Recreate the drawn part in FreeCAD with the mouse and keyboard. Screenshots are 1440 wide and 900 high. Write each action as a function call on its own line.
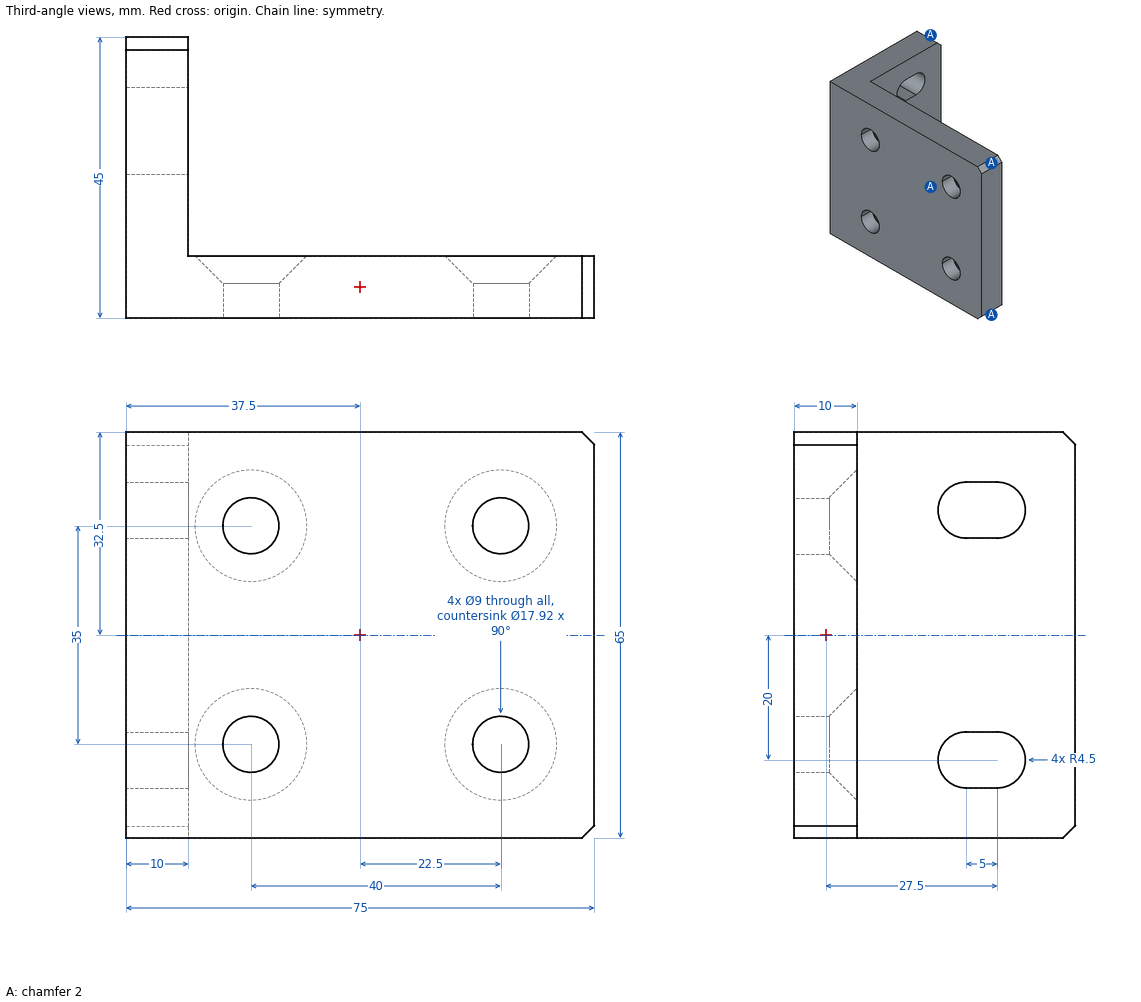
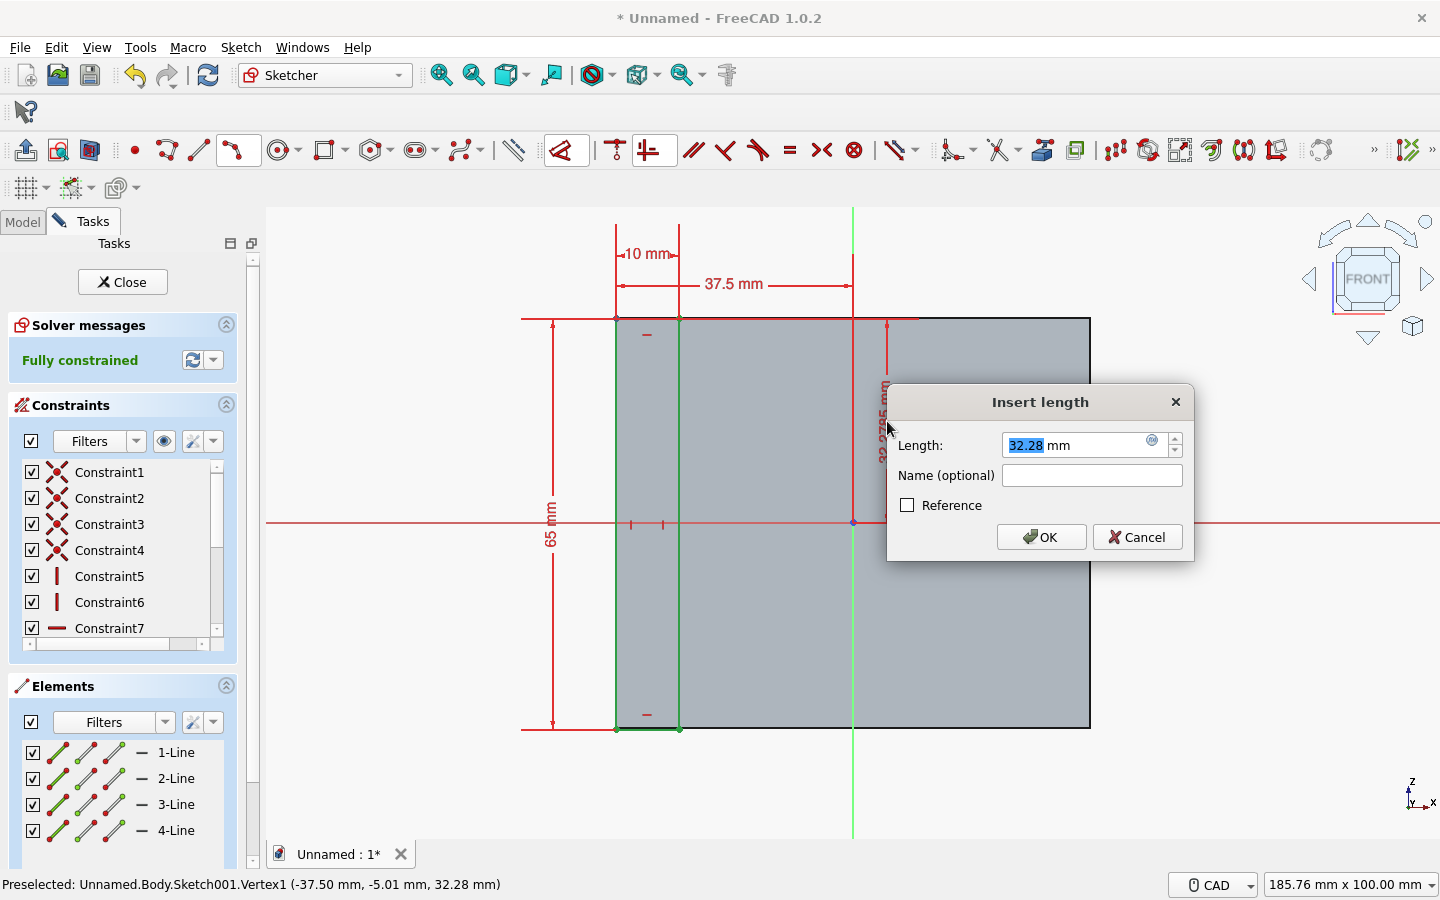
text(32.5)
key(Return)
key(Escape)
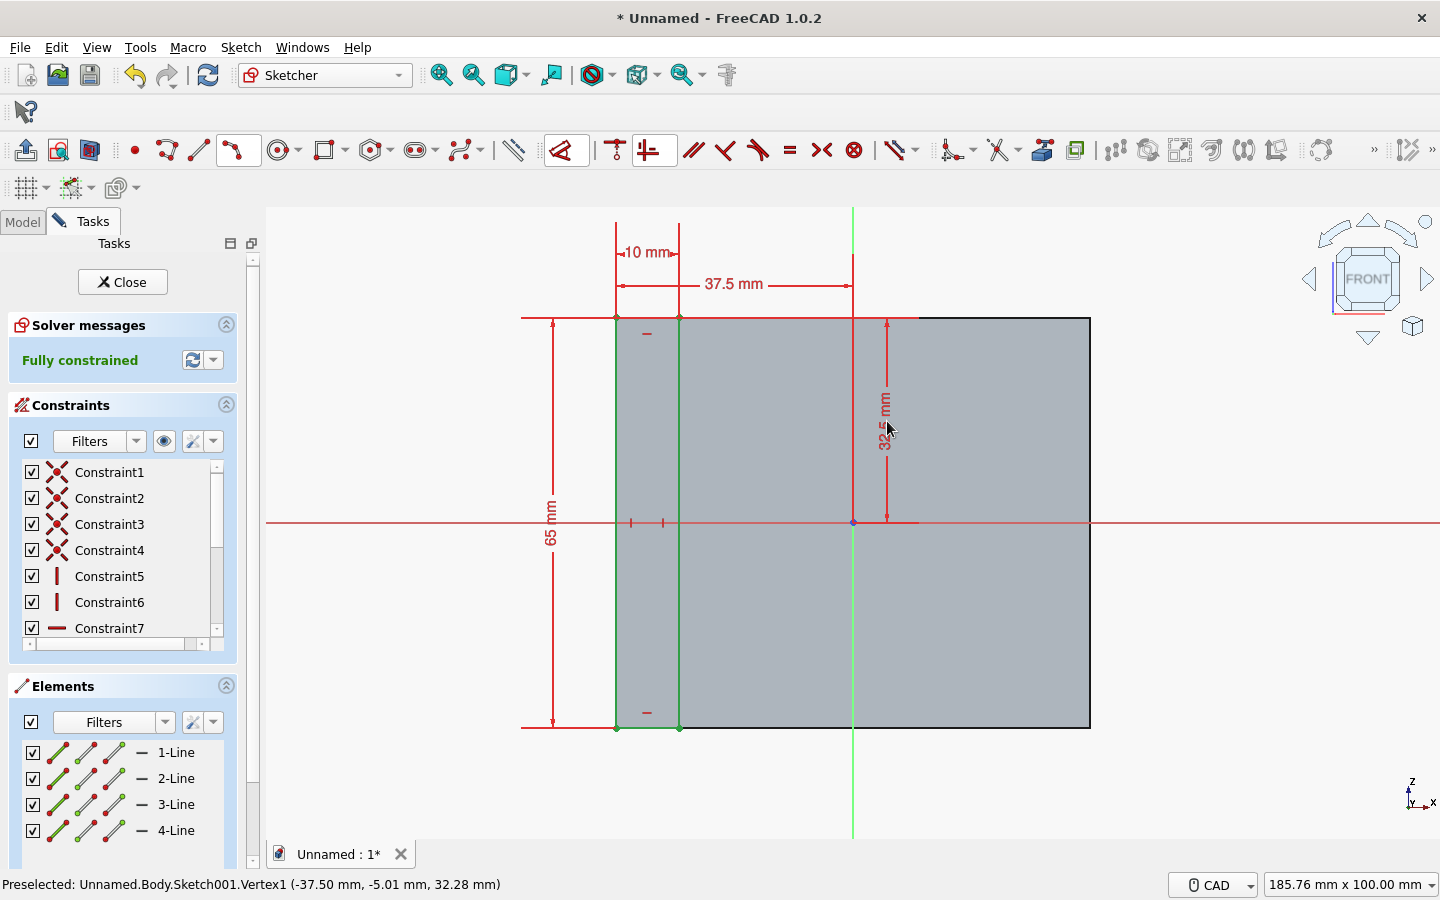
click(123, 282)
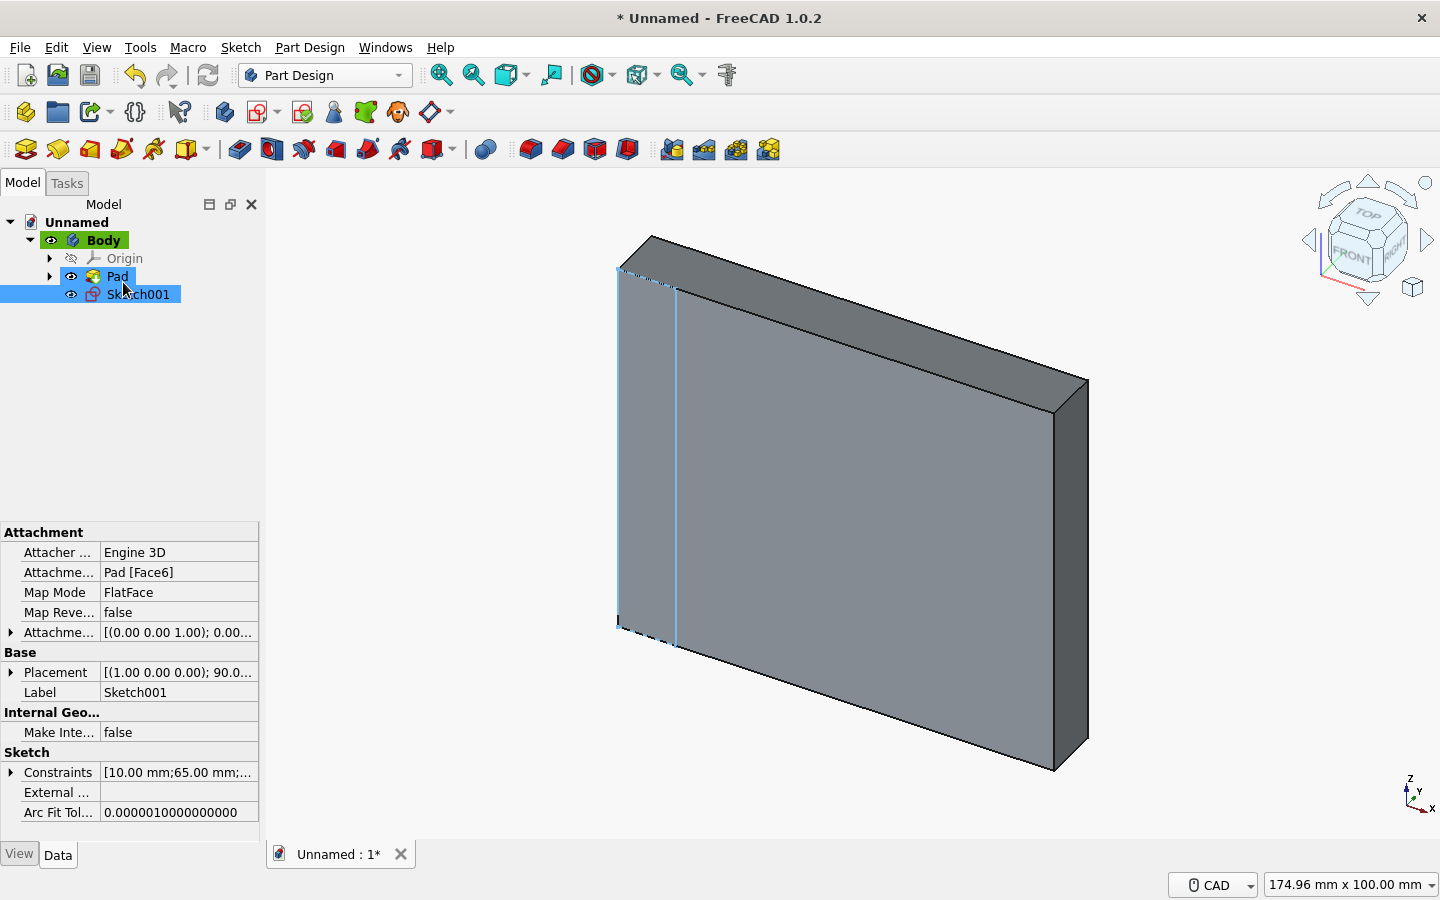
click(26, 150)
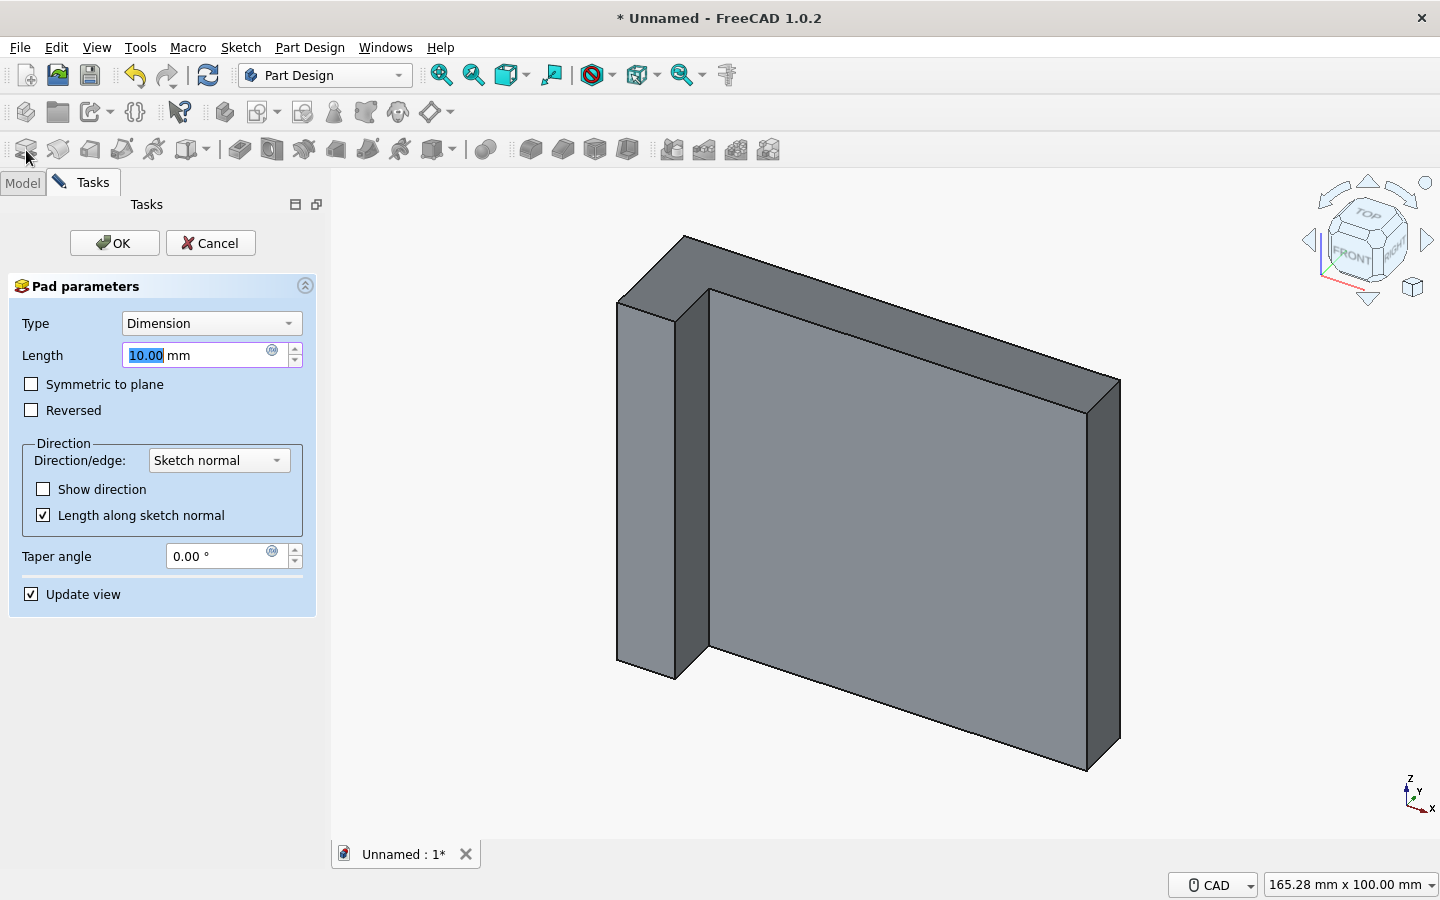
text(45)
key(Tab)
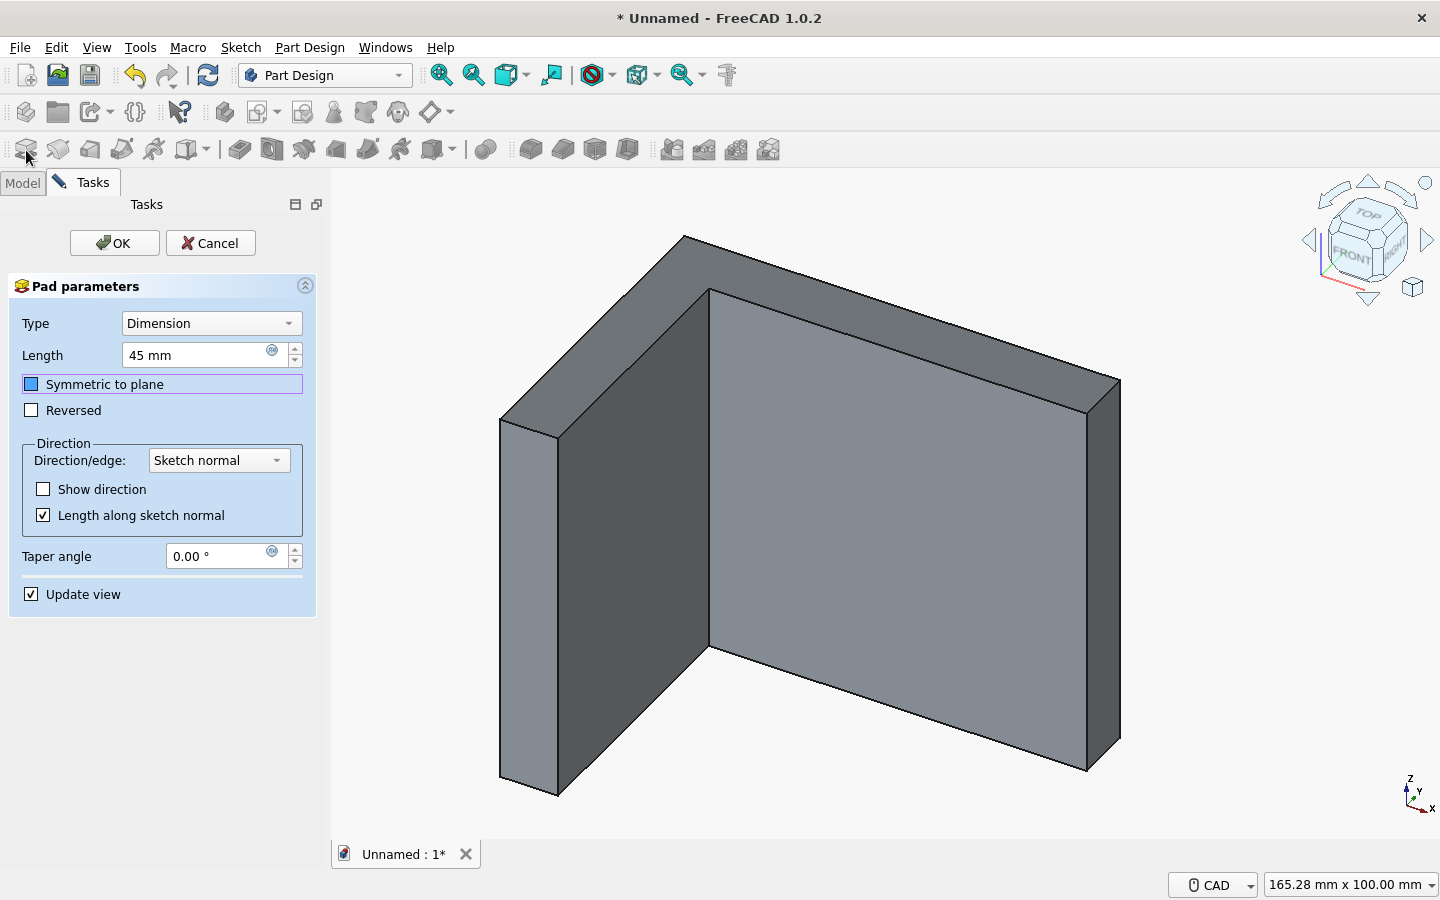
click(30, 410)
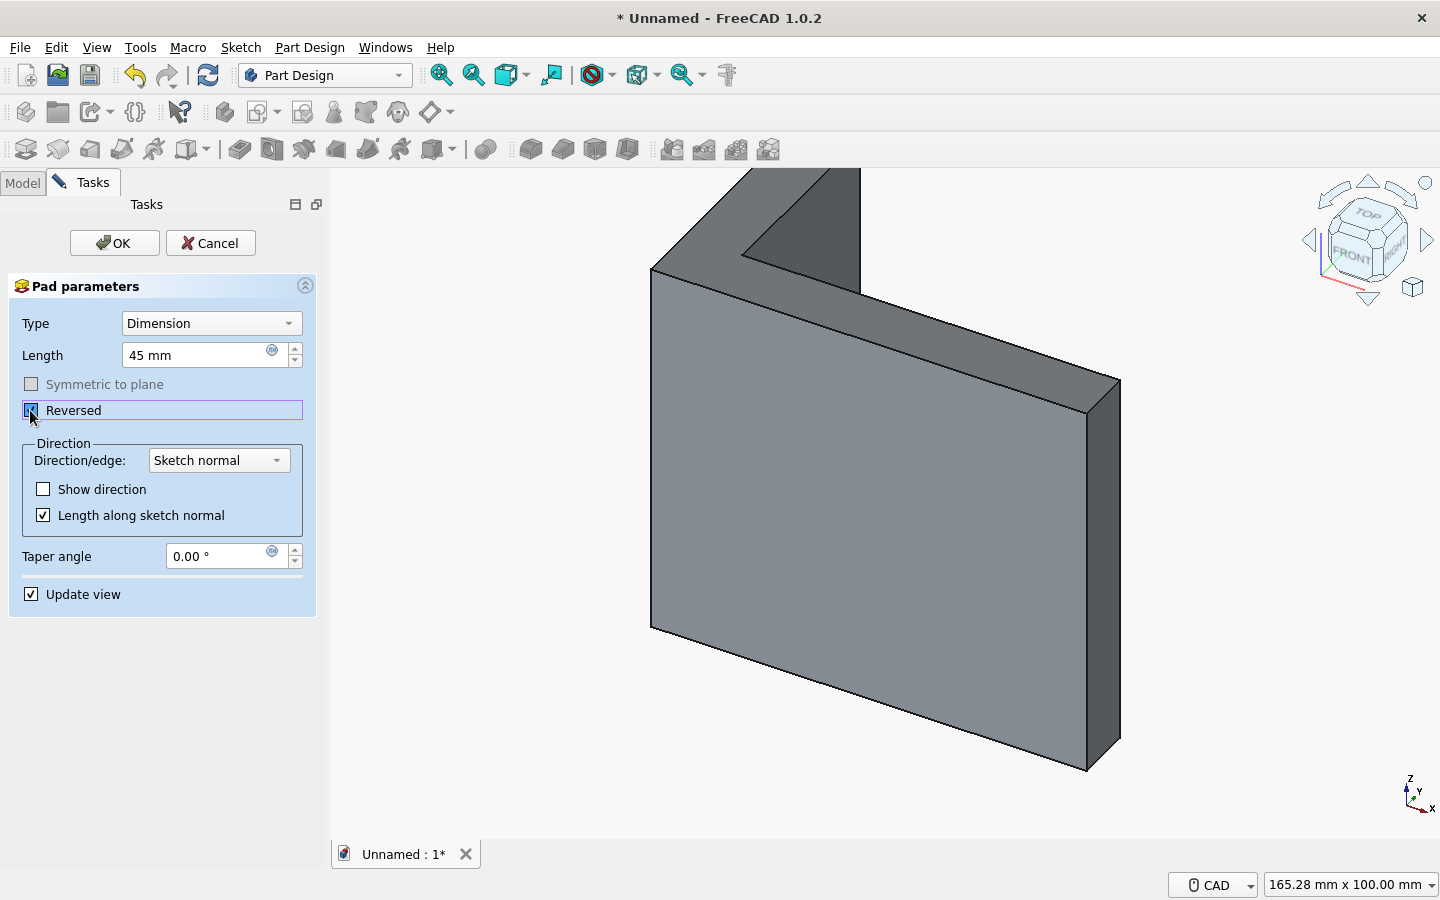
click(115, 243)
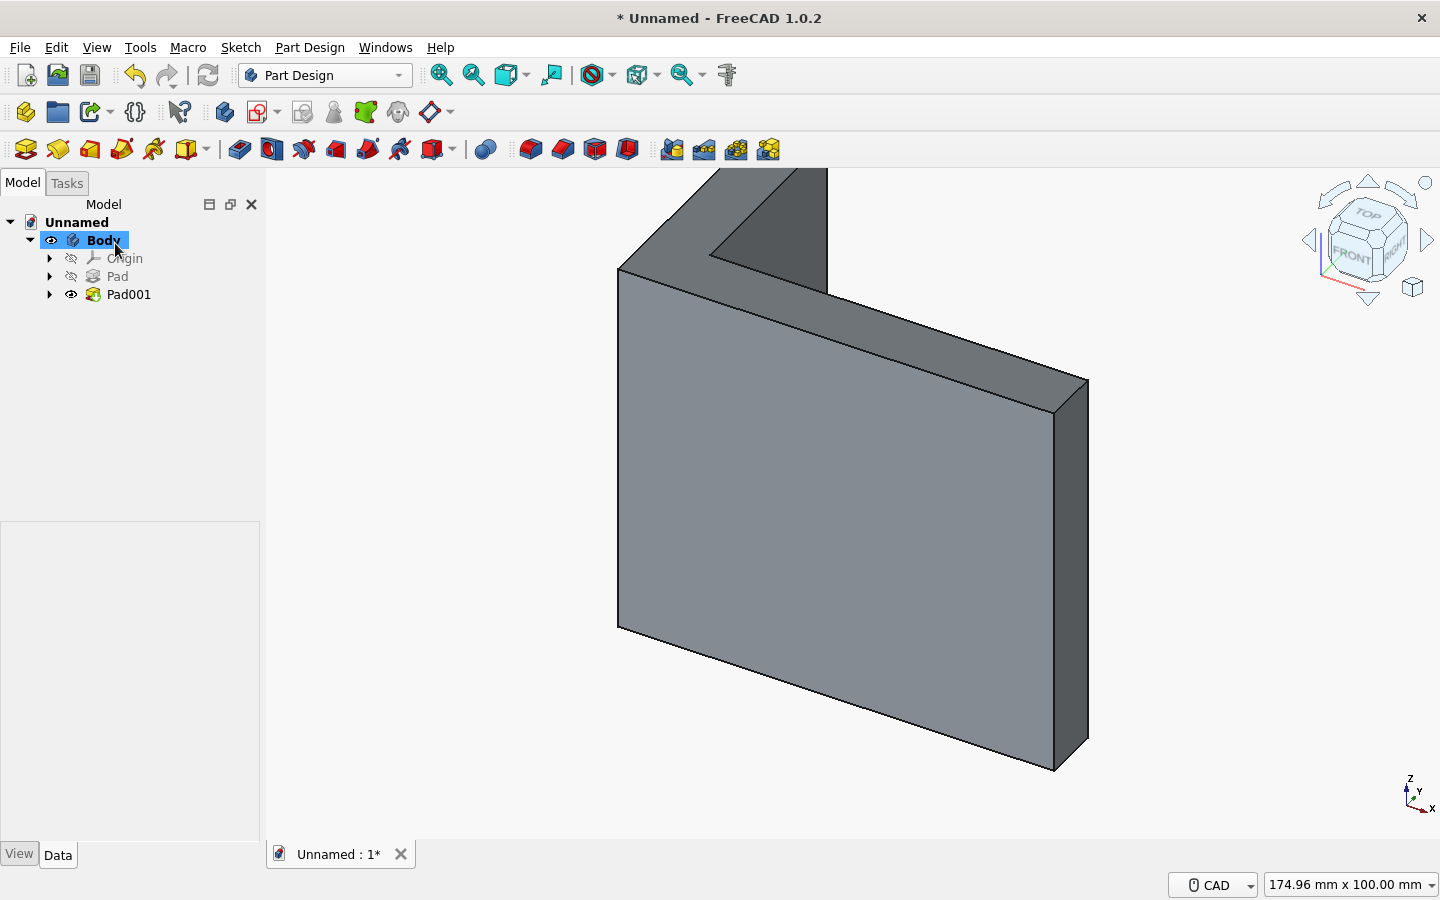
key(v)
key(f)